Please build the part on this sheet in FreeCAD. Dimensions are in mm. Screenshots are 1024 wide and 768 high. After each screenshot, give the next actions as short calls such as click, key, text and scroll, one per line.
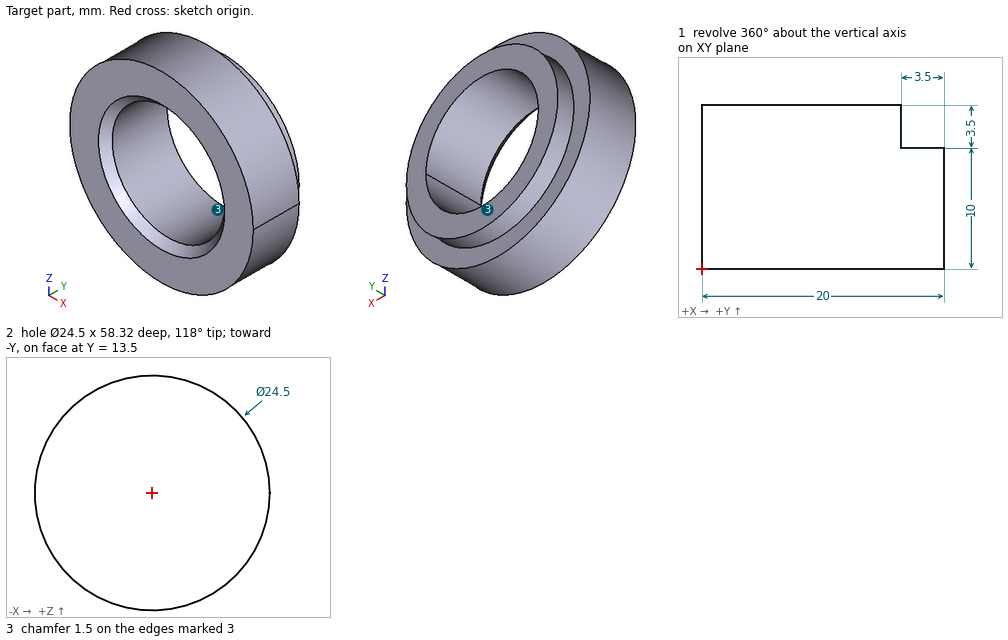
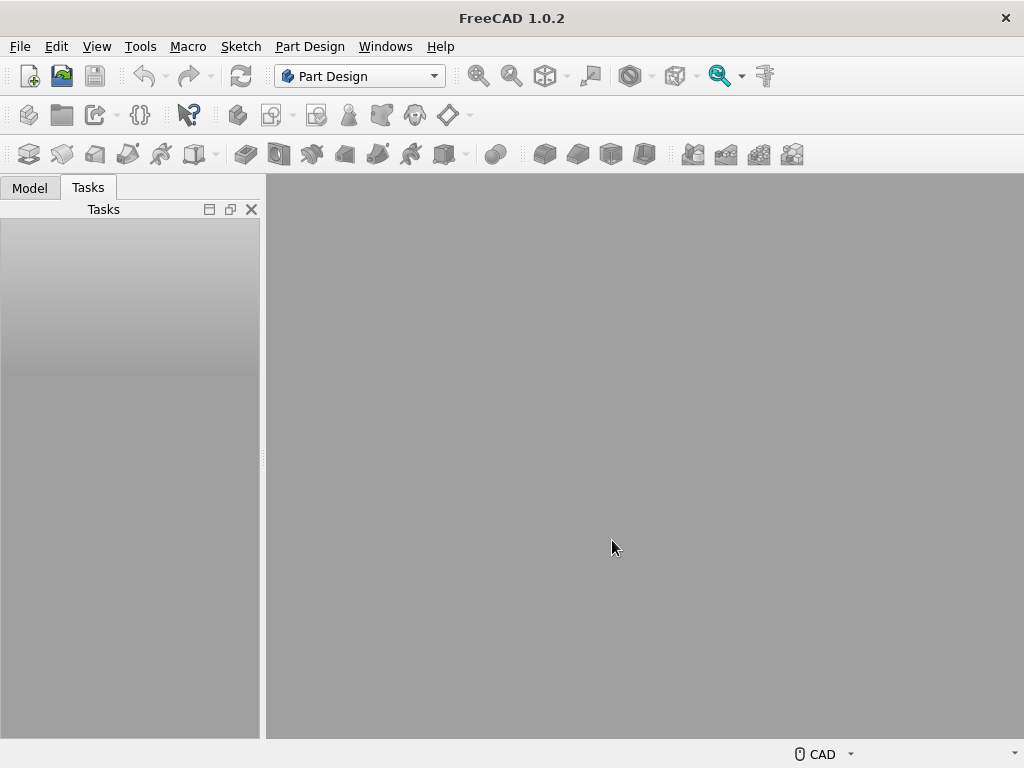
click(29, 76)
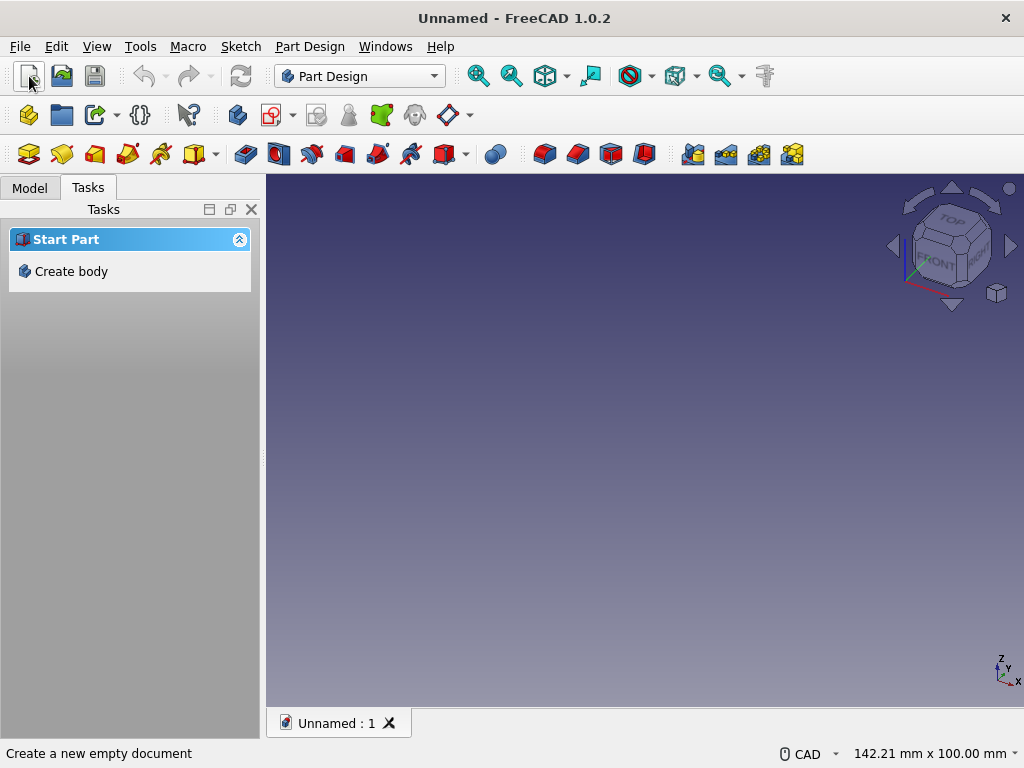
click(270, 116)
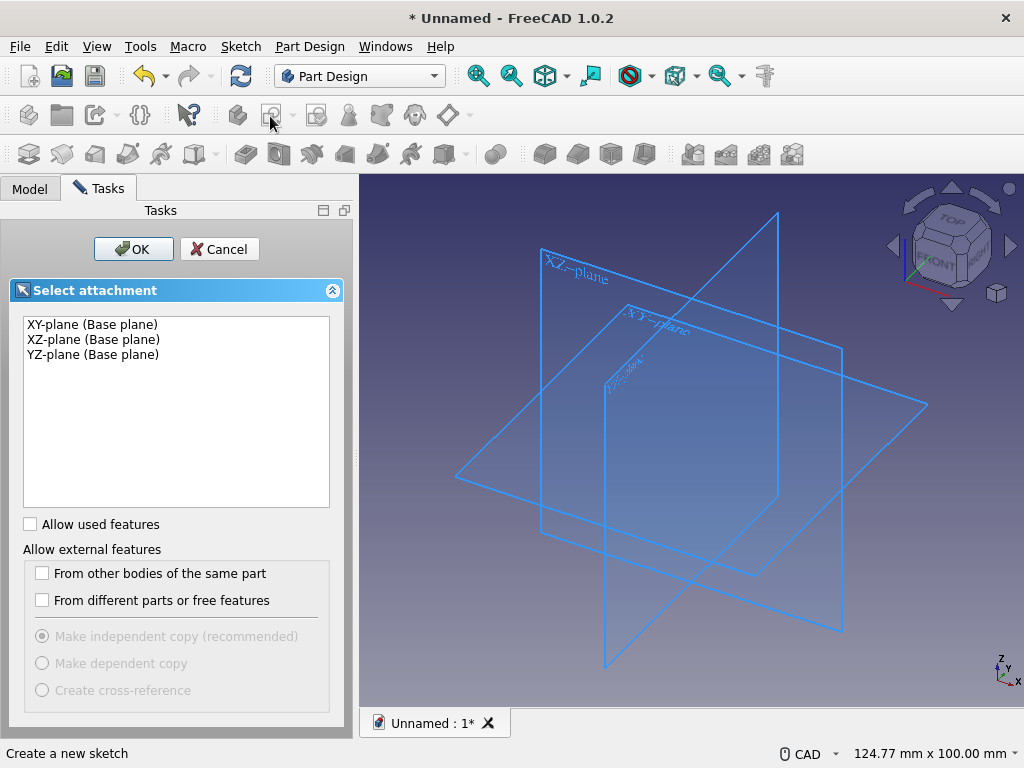
click(84, 324)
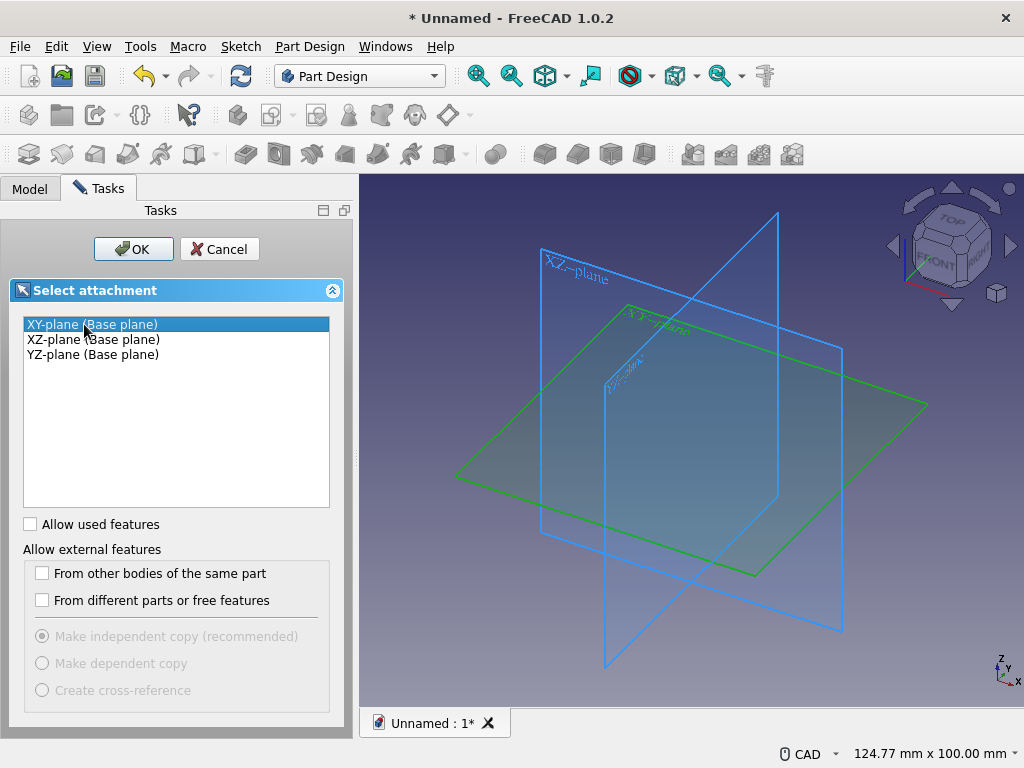
click(134, 249)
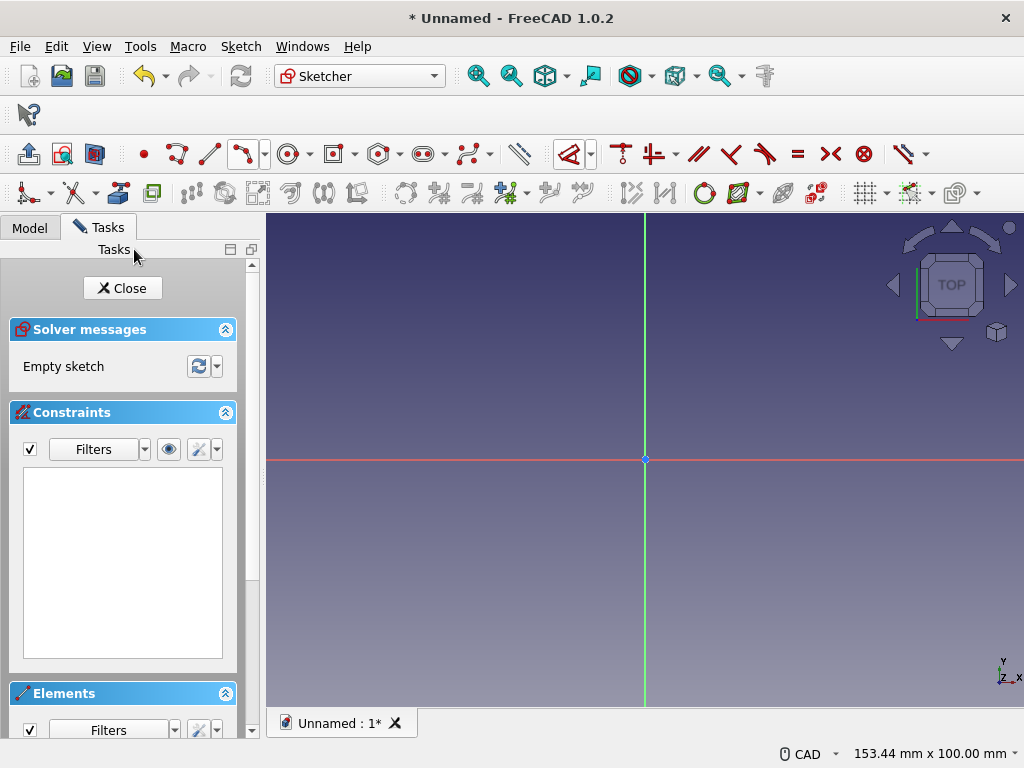
scroll(733, 416, up, 7)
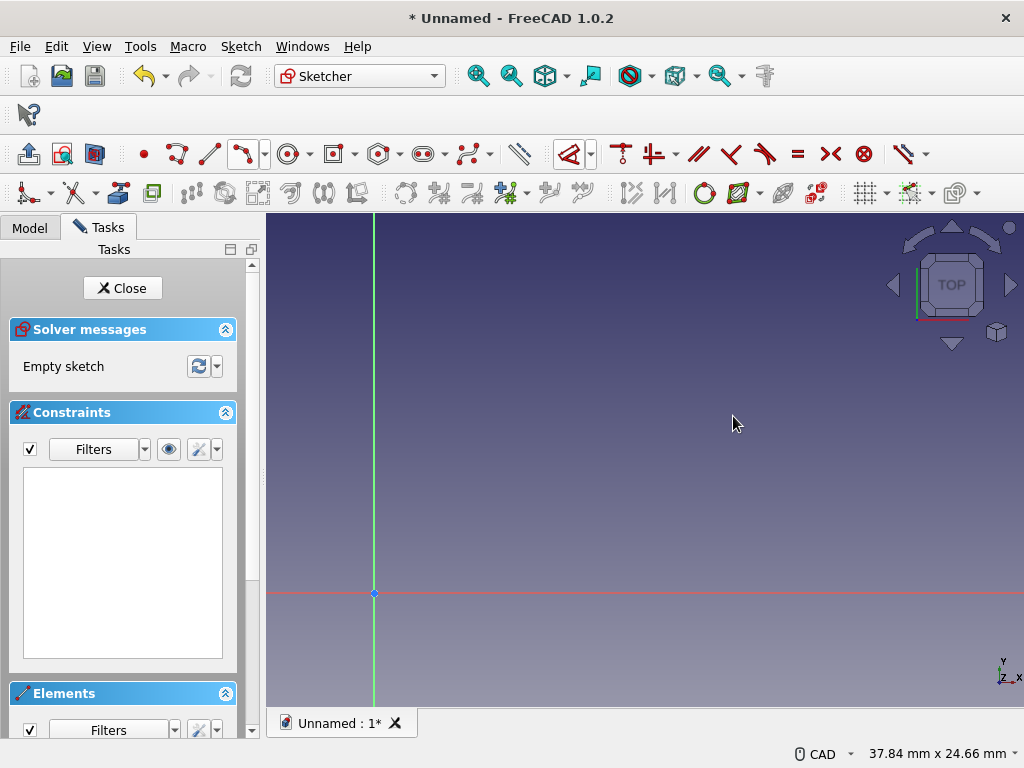
click(177, 154)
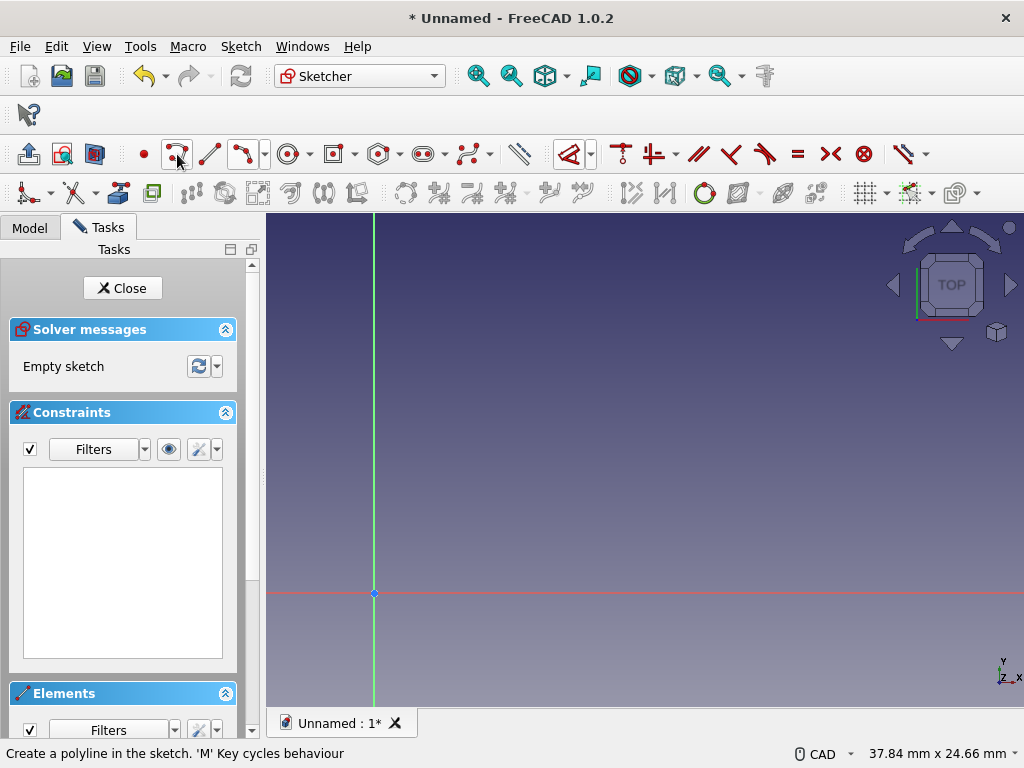
click(374, 593)
click(775, 584)
click(775, 393)
click(705, 393)
click(705, 323)
click(383, 323)
click(374, 593)
key(Escape)
key(Escape)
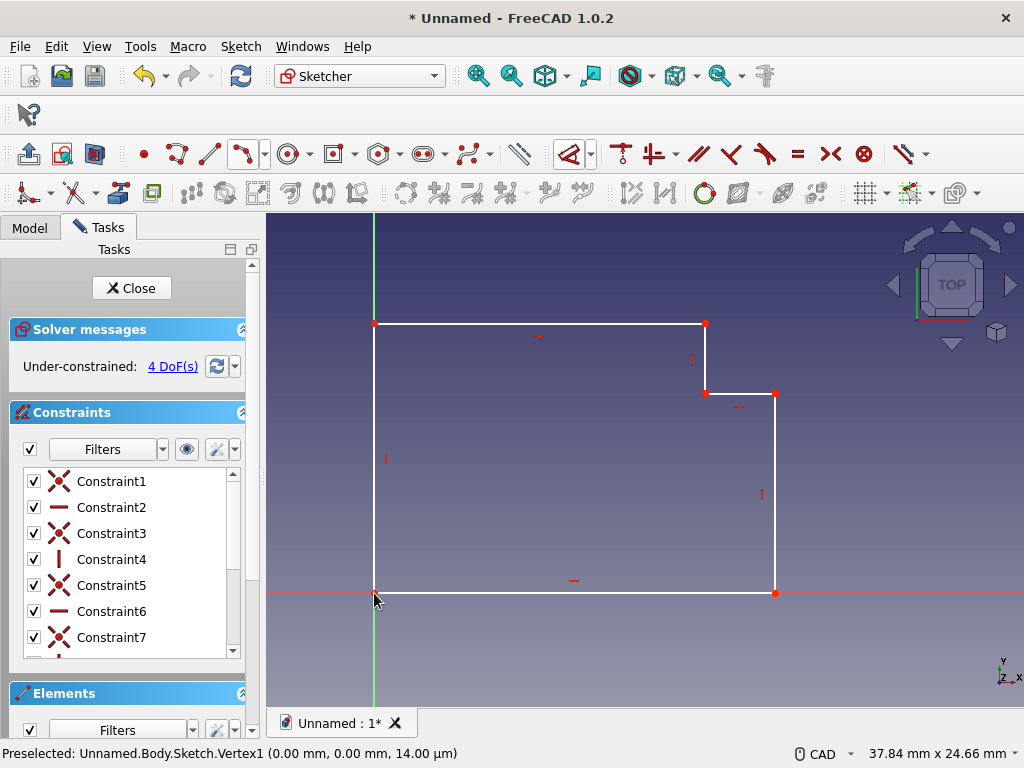
click(568, 154)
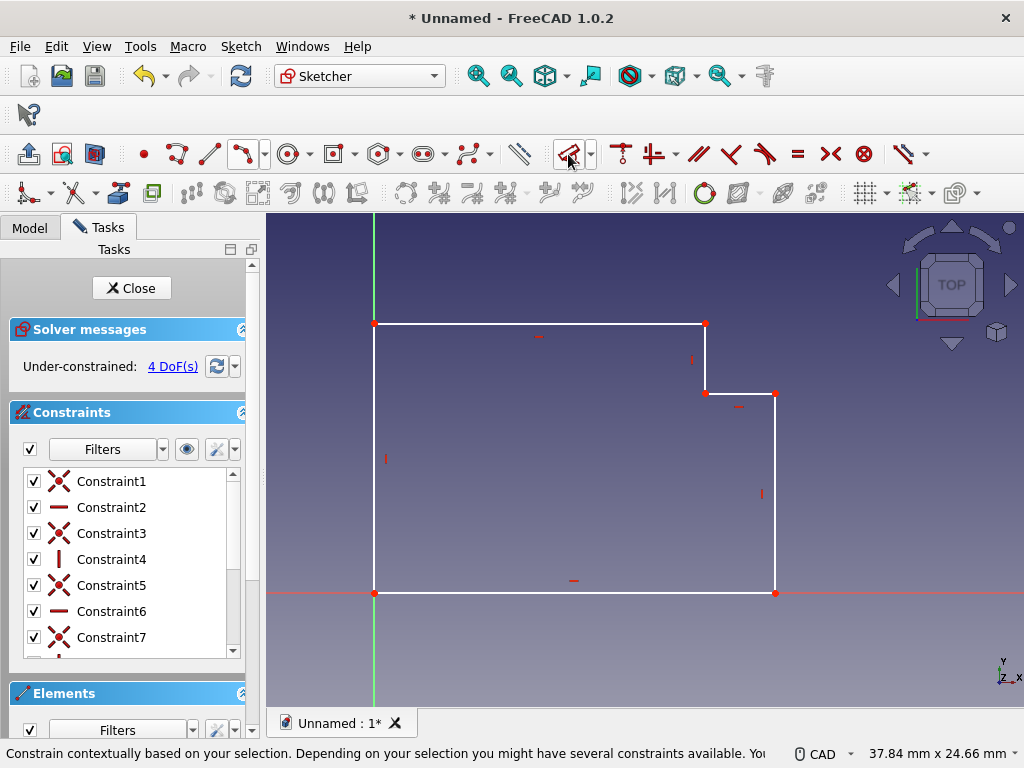
click(494, 593)
click(575, 627)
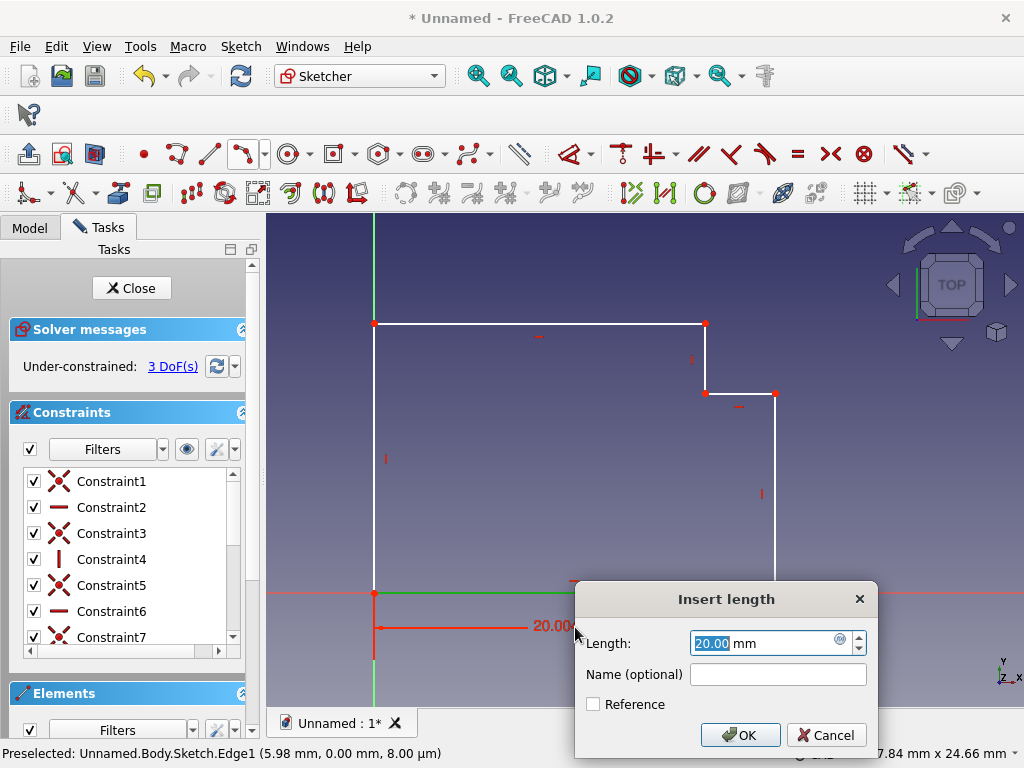
text(20)
key(Return)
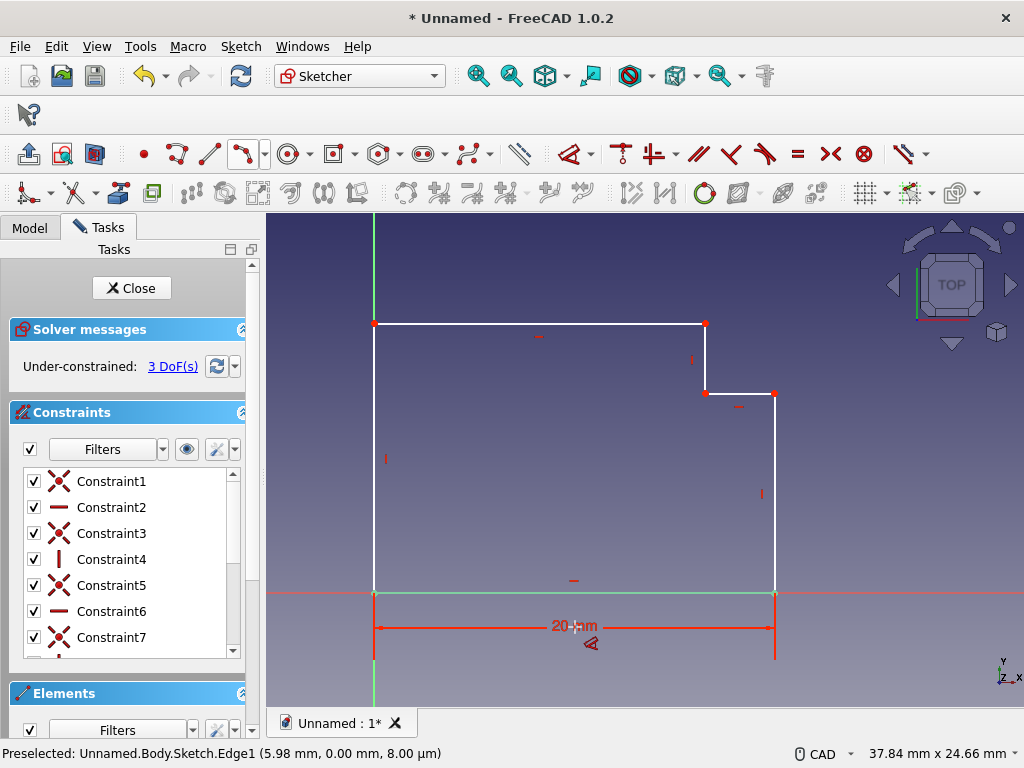
click(775, 533)
click(809, 494)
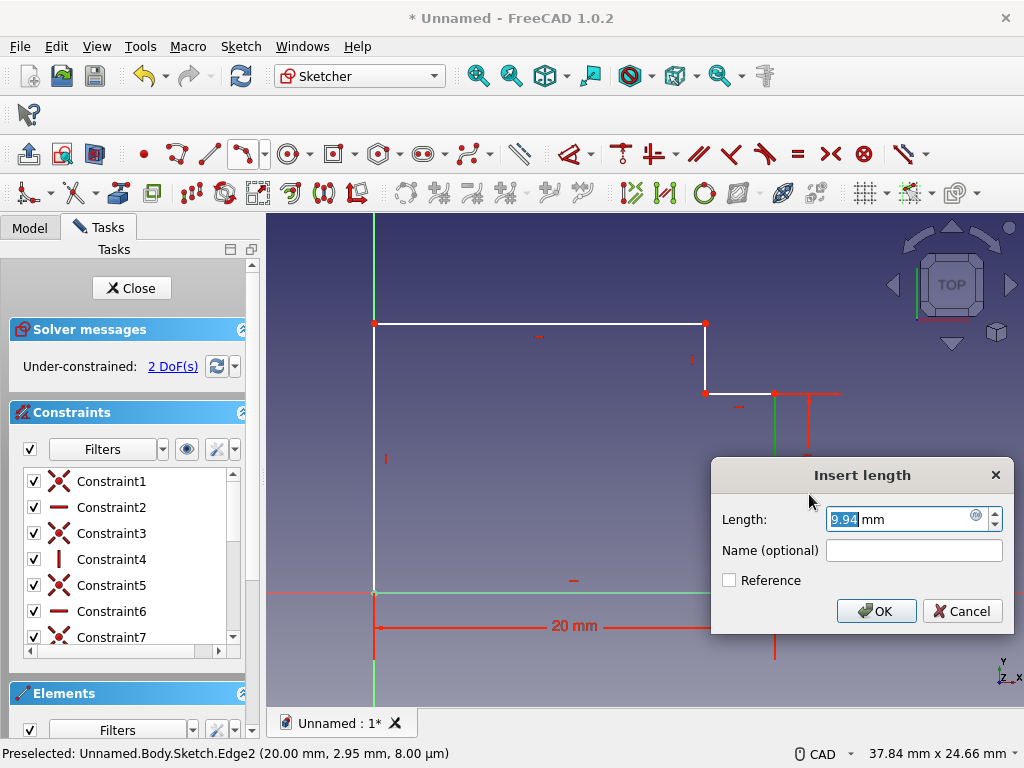
text(10)
key(Return)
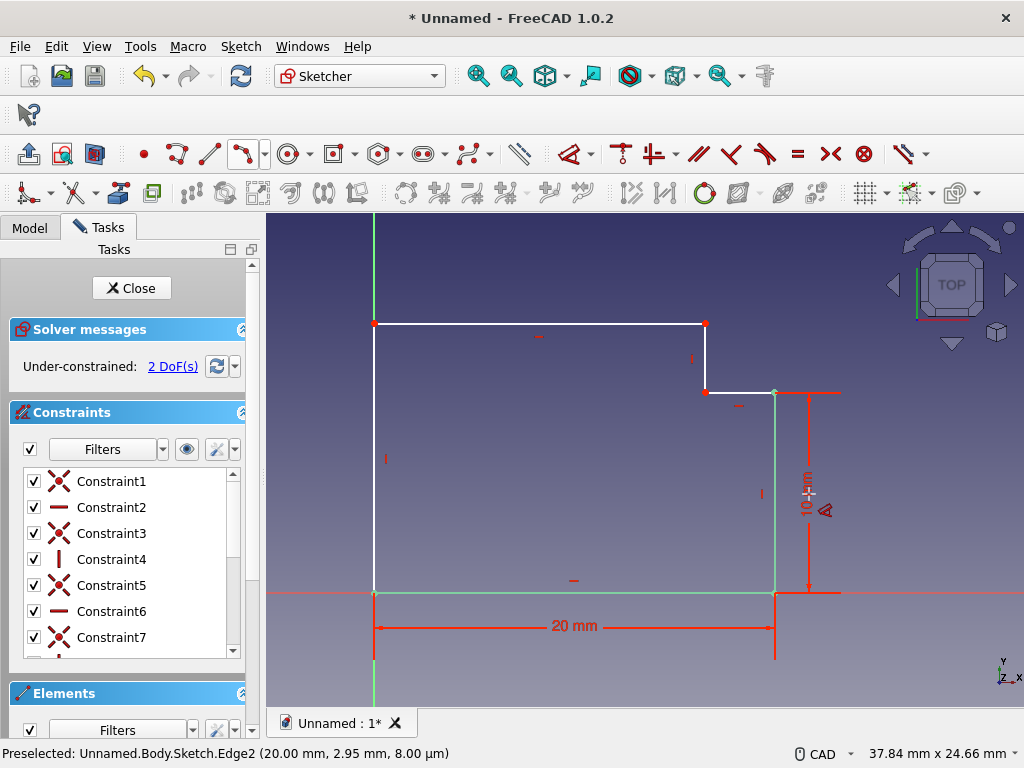
click(754, 393)
click(740, 359)